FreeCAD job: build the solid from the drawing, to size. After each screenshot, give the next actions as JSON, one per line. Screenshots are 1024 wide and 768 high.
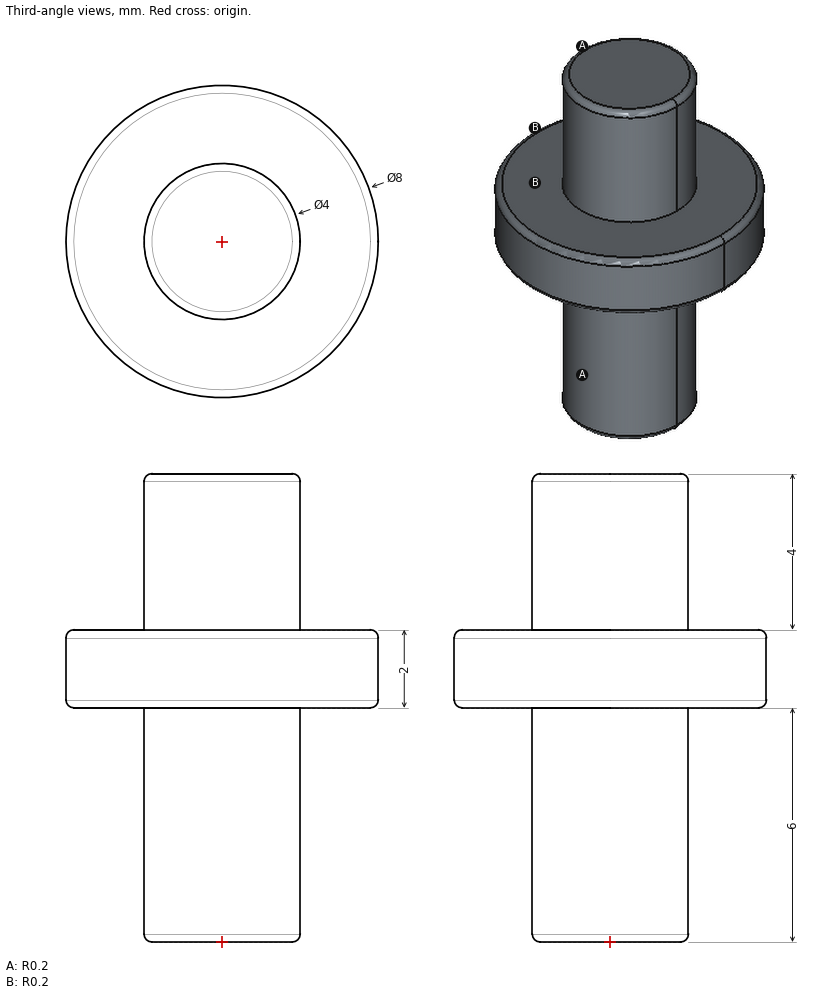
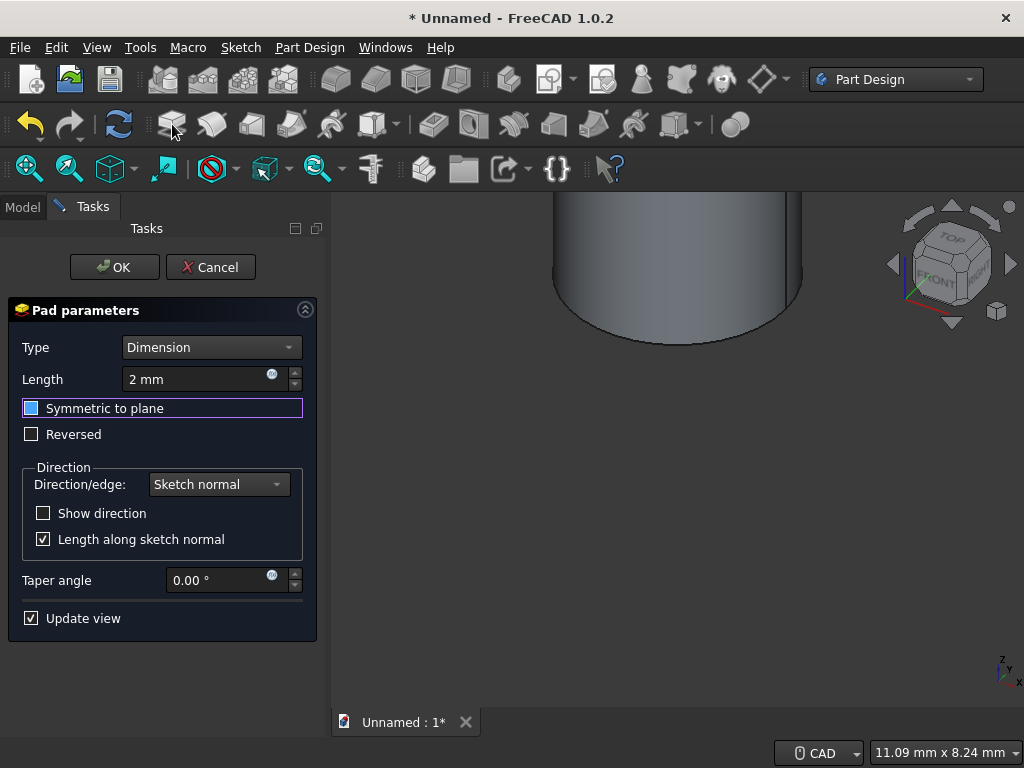
{"action": "left_click", "coordinate": [115, 267]}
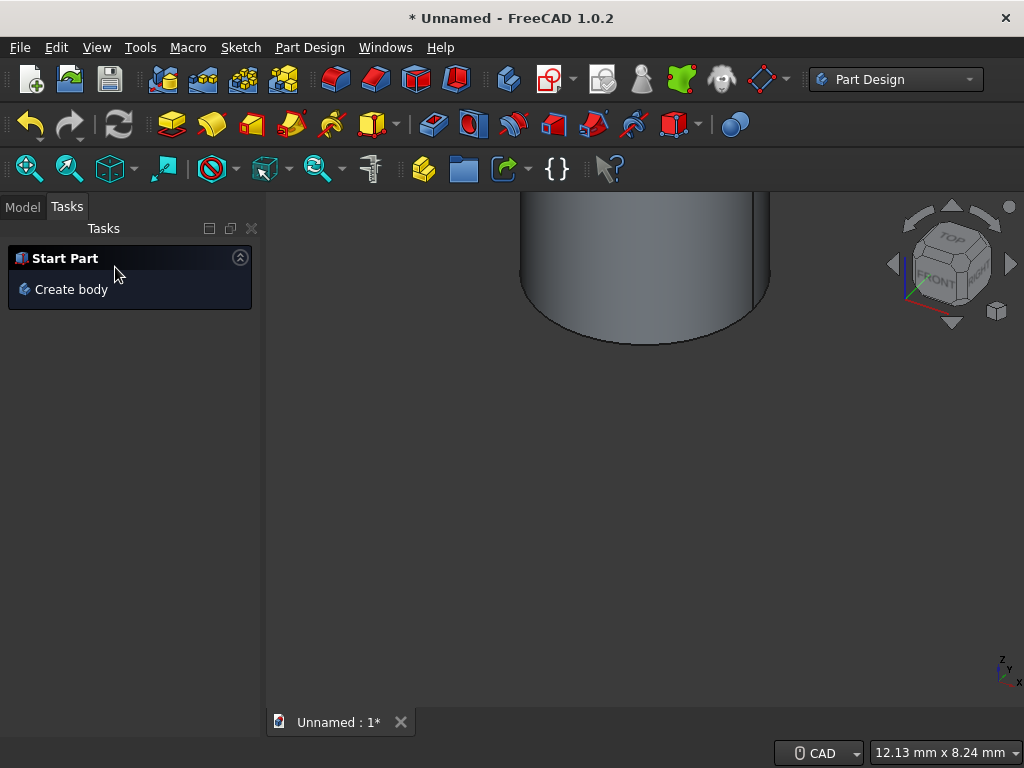
{"action": "left_click", "coordinate": [30, 170]}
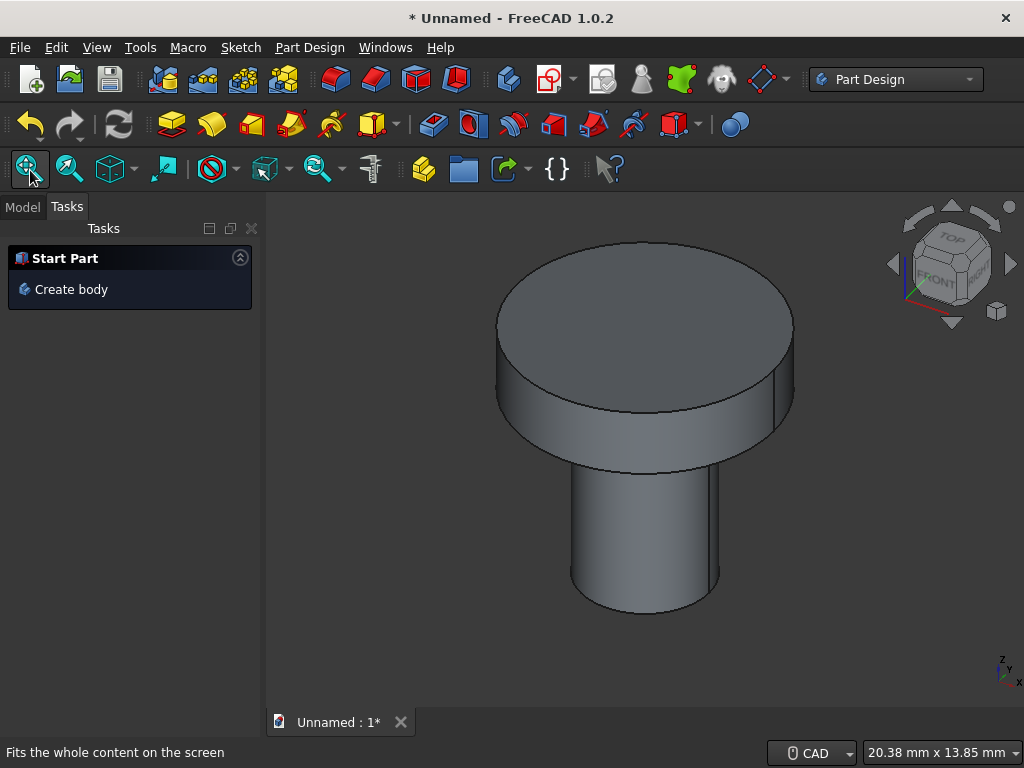
{"action": "left_click", "coordinate": [645, 327]}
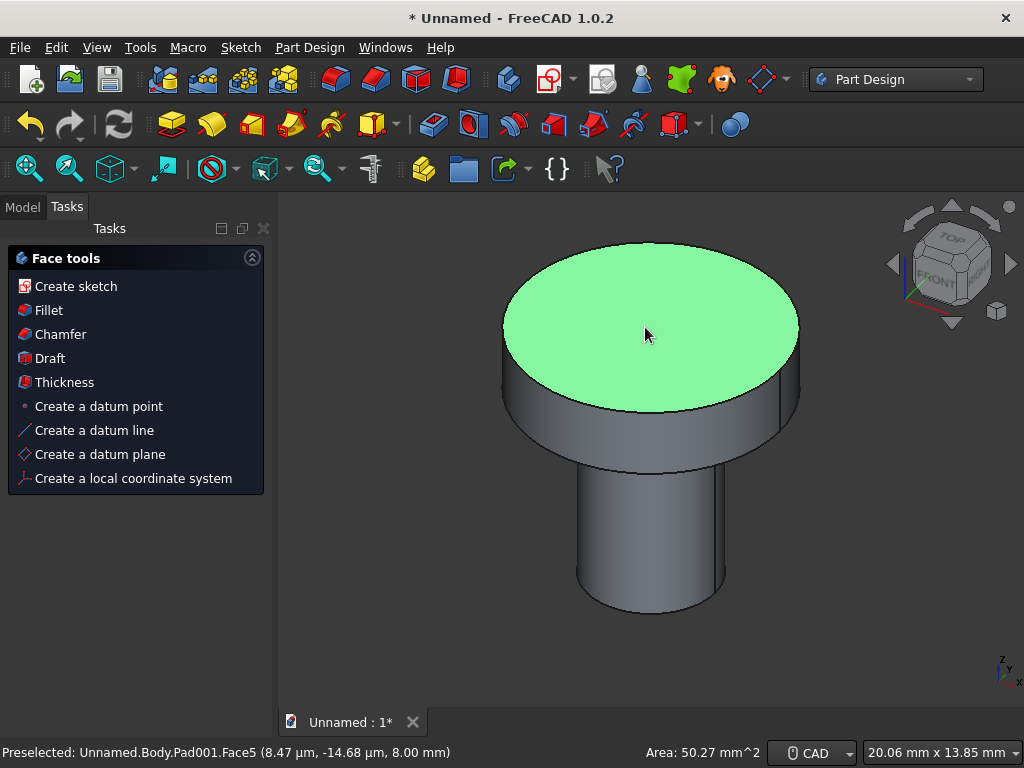
{"action": "left_click", "coordinate": [550, 80]}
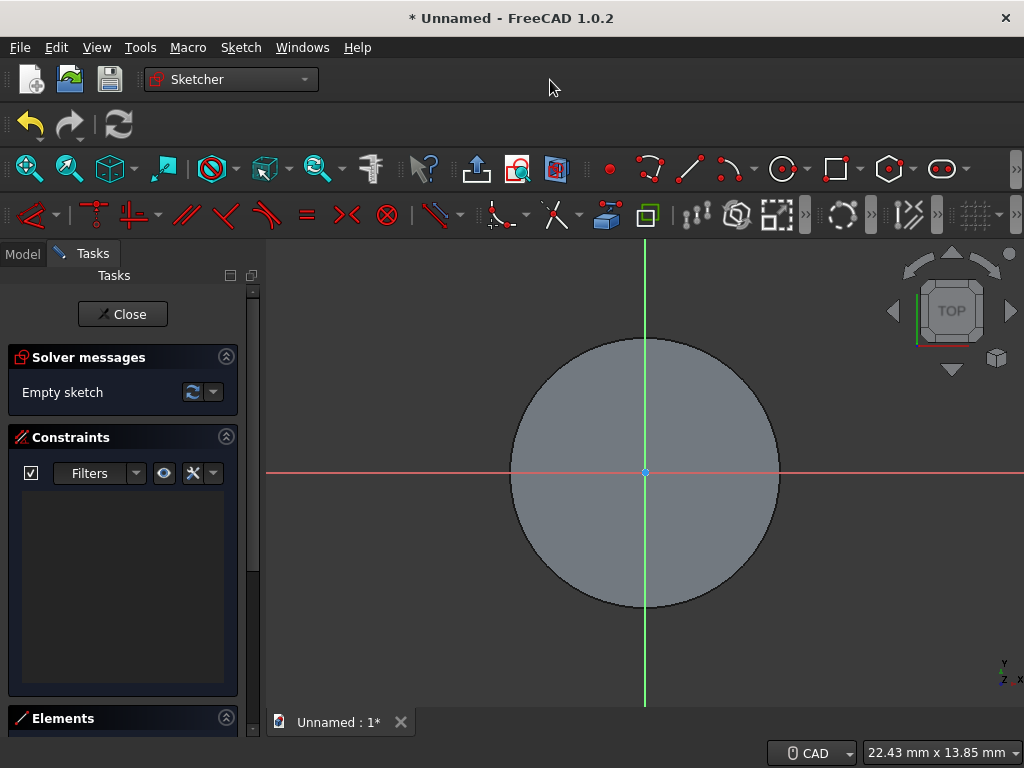
{"action": "scroll", "coordinate": [701, 473], "scroll_direction": "up", "scroll_amount": 4}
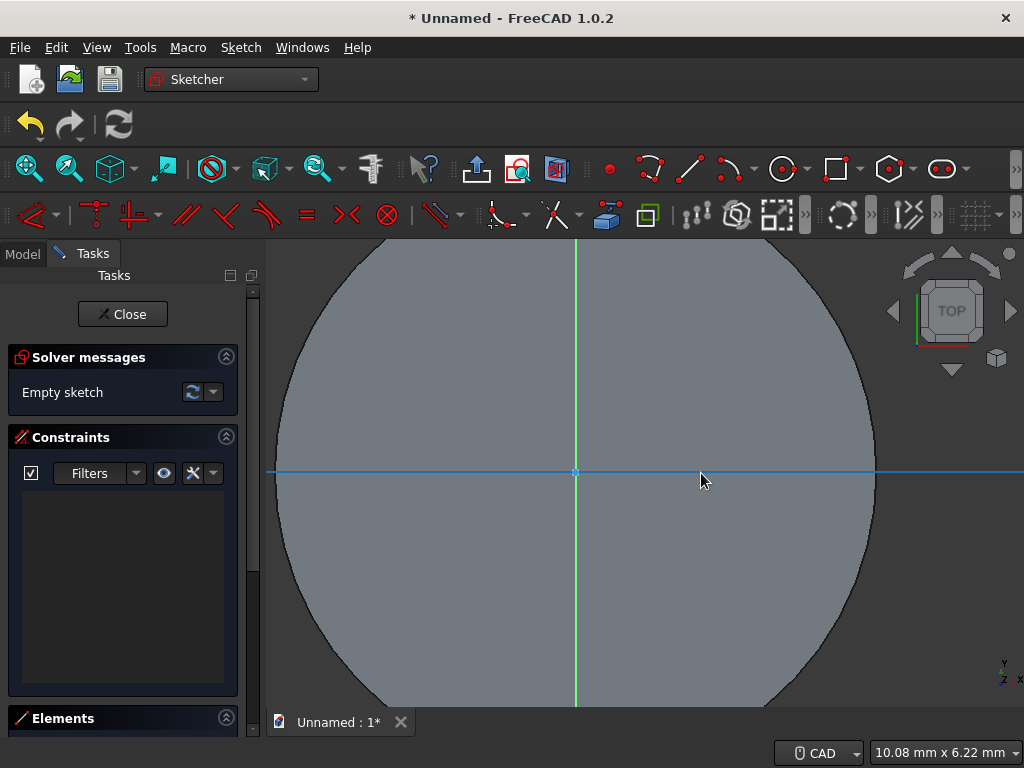
{"action": "left_click", "coordinate": [784, 170]}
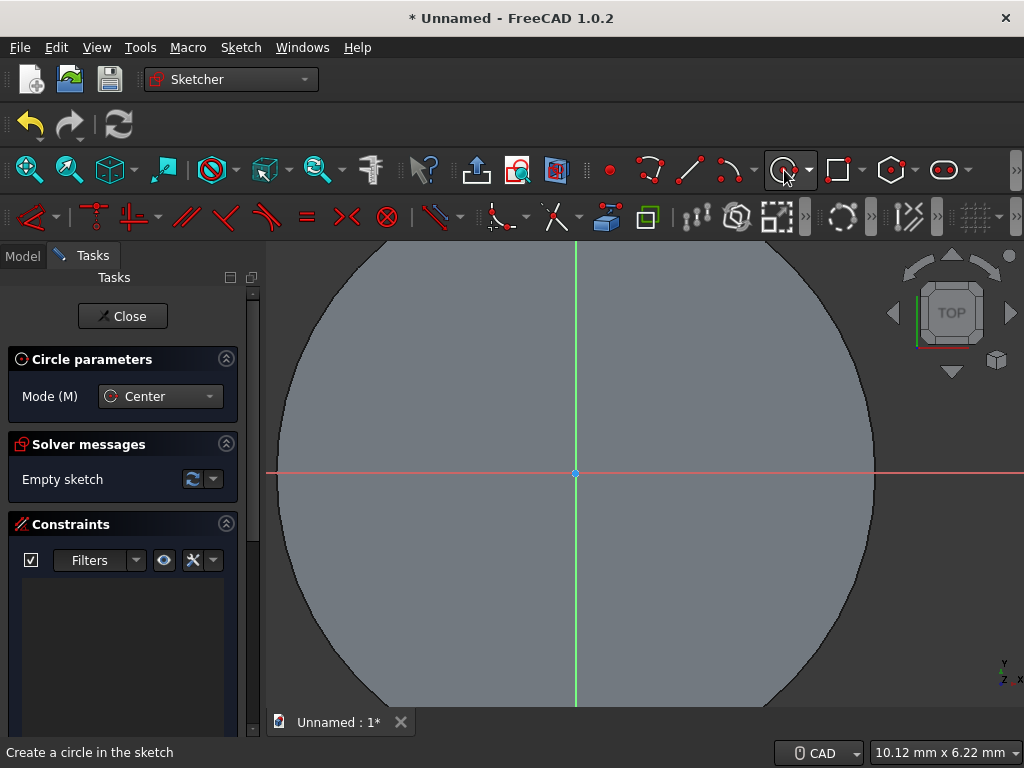
{"action": "left_click", "coordinate": [576, 473]}
{"action": "left_click", "coordinate": [682, 367]}
{"action": "key", "text": "Escape"}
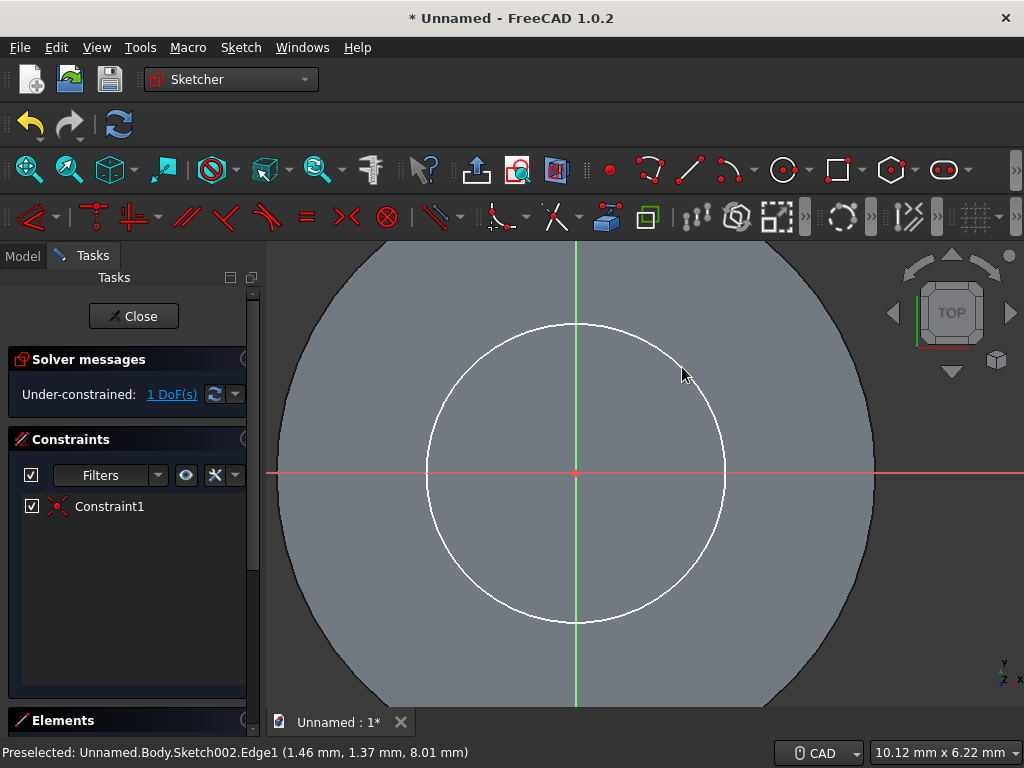
{"action": "left_click", "coordinate": [32, 218]}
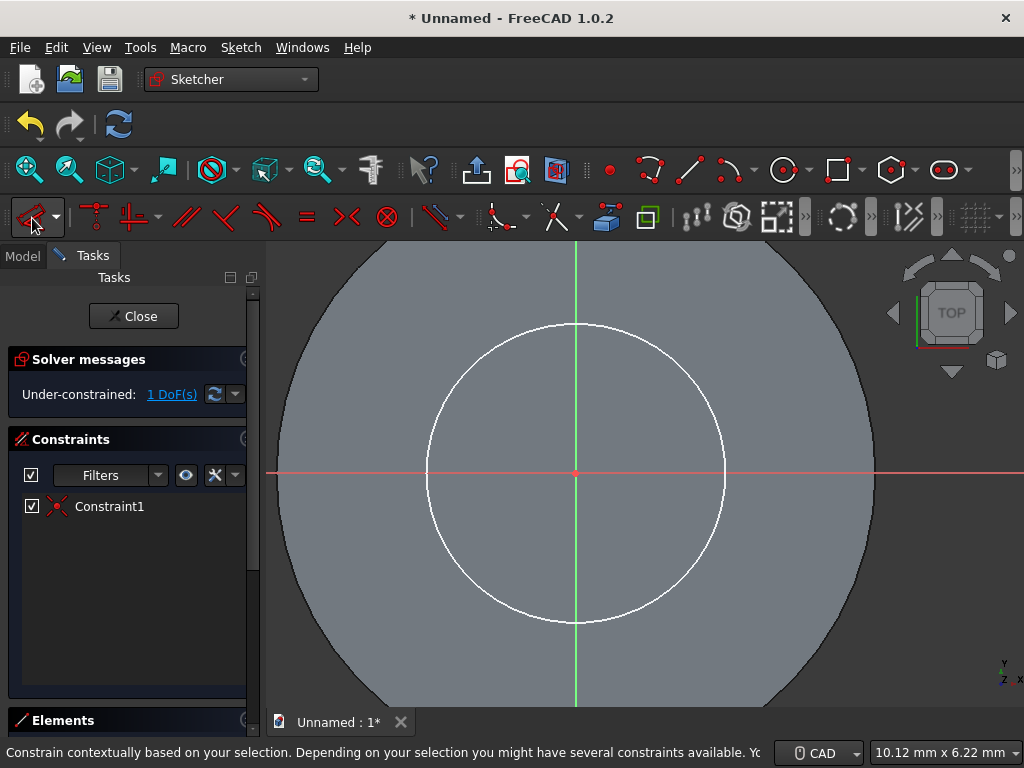
{"action": "left_click", "coordinate": [681, 367]}
{"action": "left_click", "coordinate": [703, 344]}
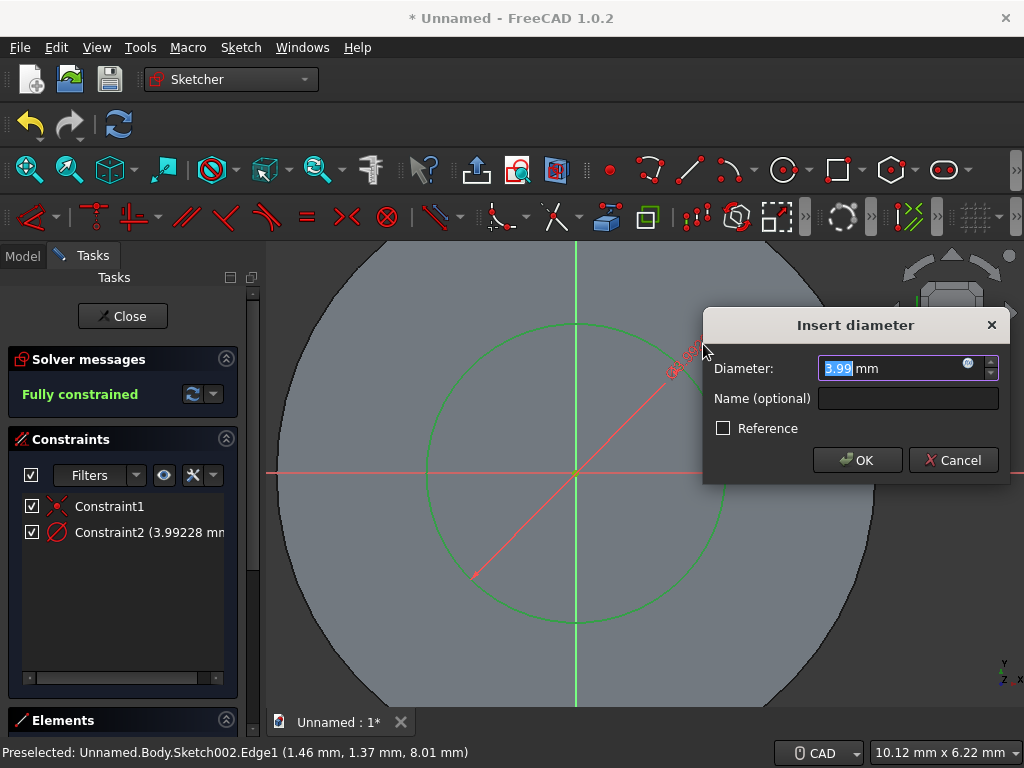
{"action": "type", "text": "4"}
{"action": "key", "text": "Return"}
{"action": "key", "text": "Escape"}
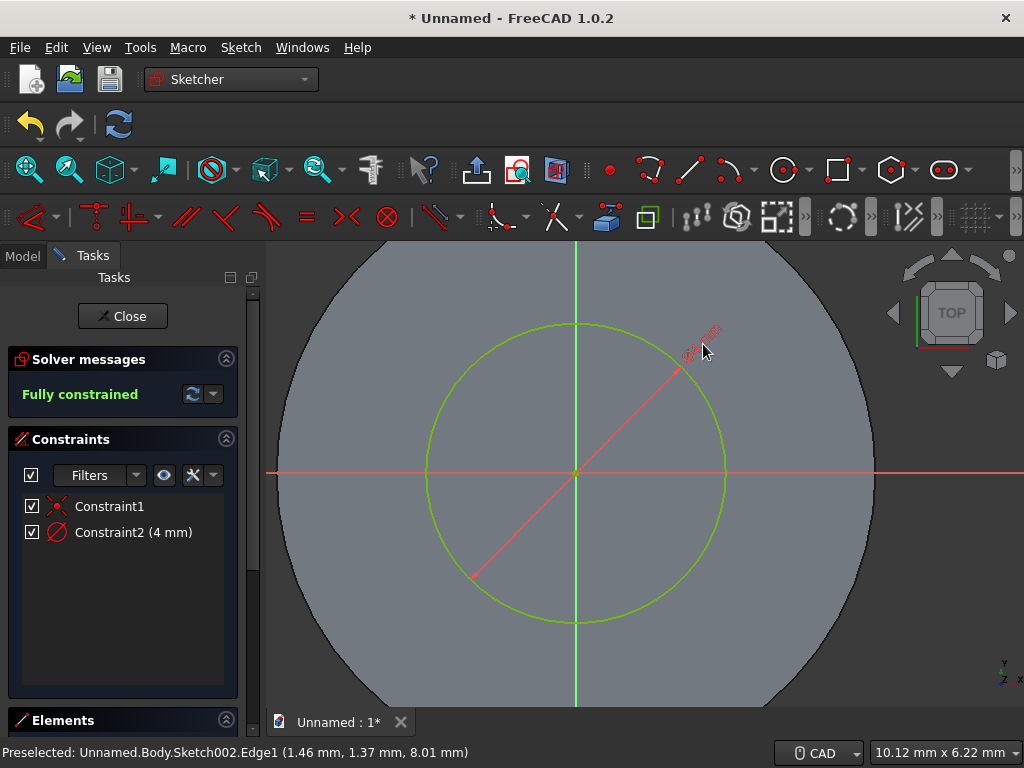
{"action": "left_click", "coordinate": [123, 316]}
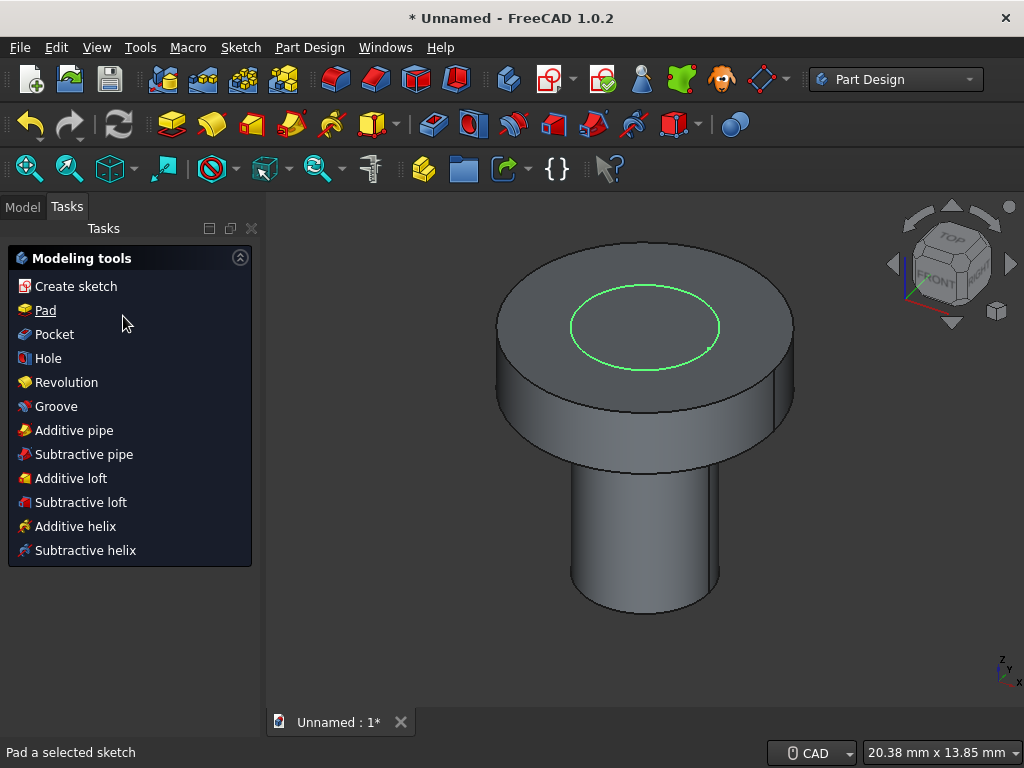
{"action": "left_click", "coordinate": [172, 124]}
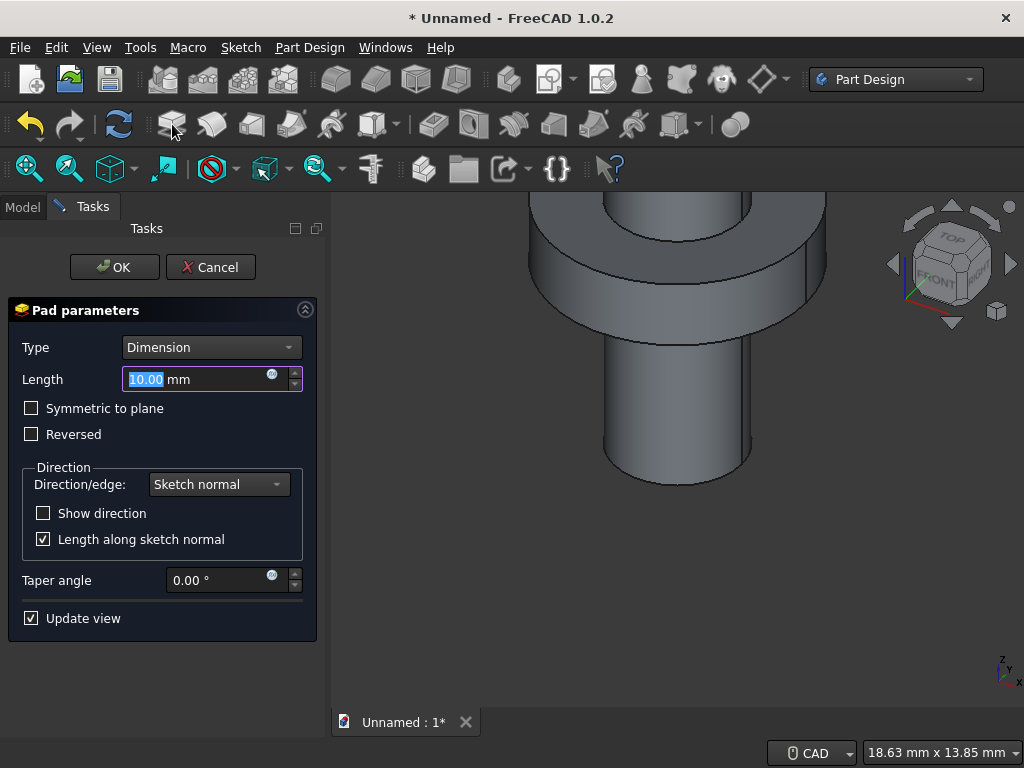
{"action": "type", "text": "4"}
{"action": "key", "text": "Tab"}